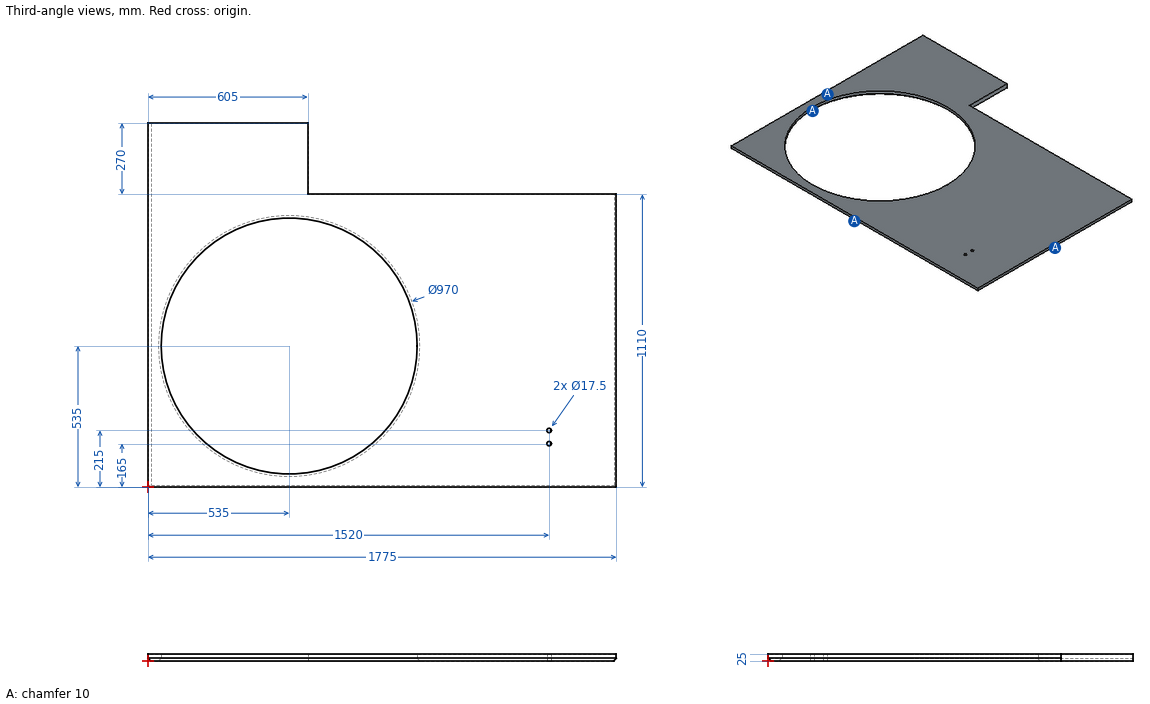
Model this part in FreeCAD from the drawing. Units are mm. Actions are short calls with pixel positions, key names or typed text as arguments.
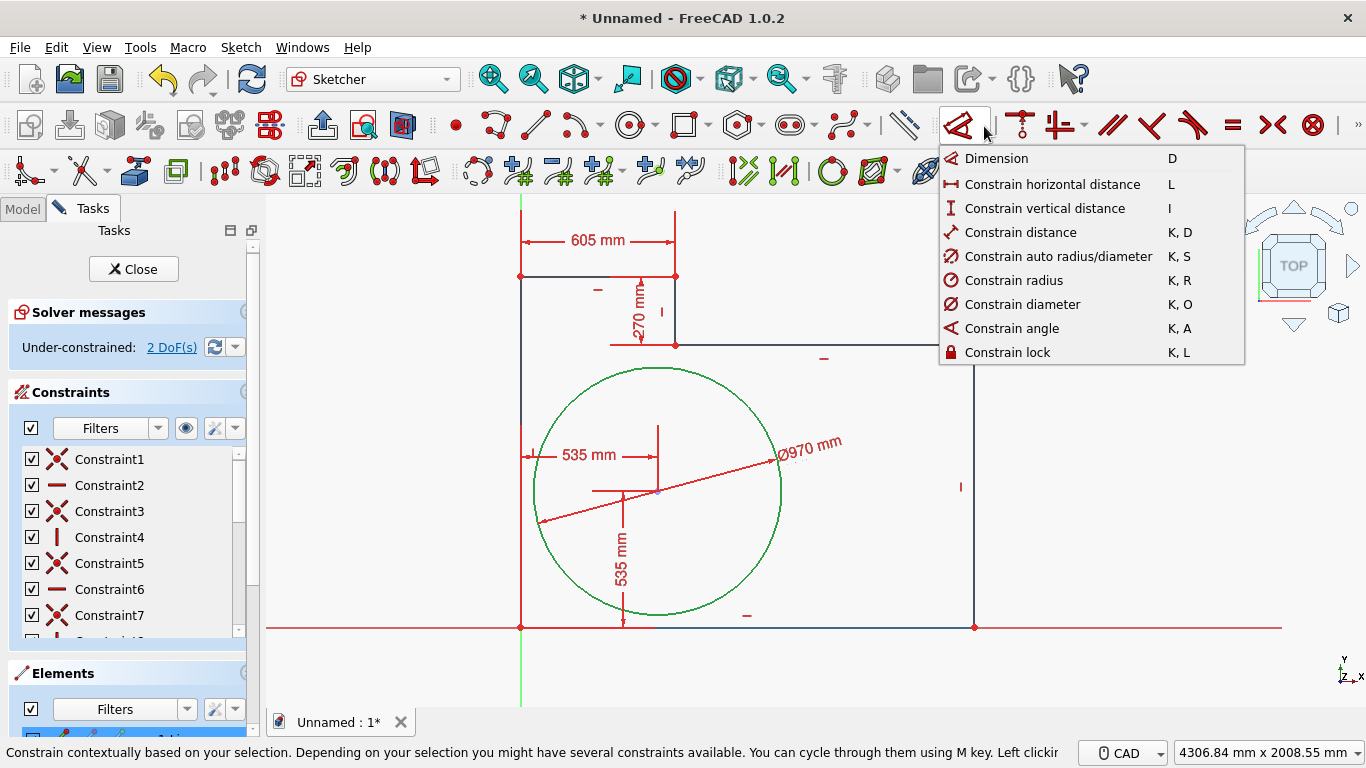
click(1092, 184)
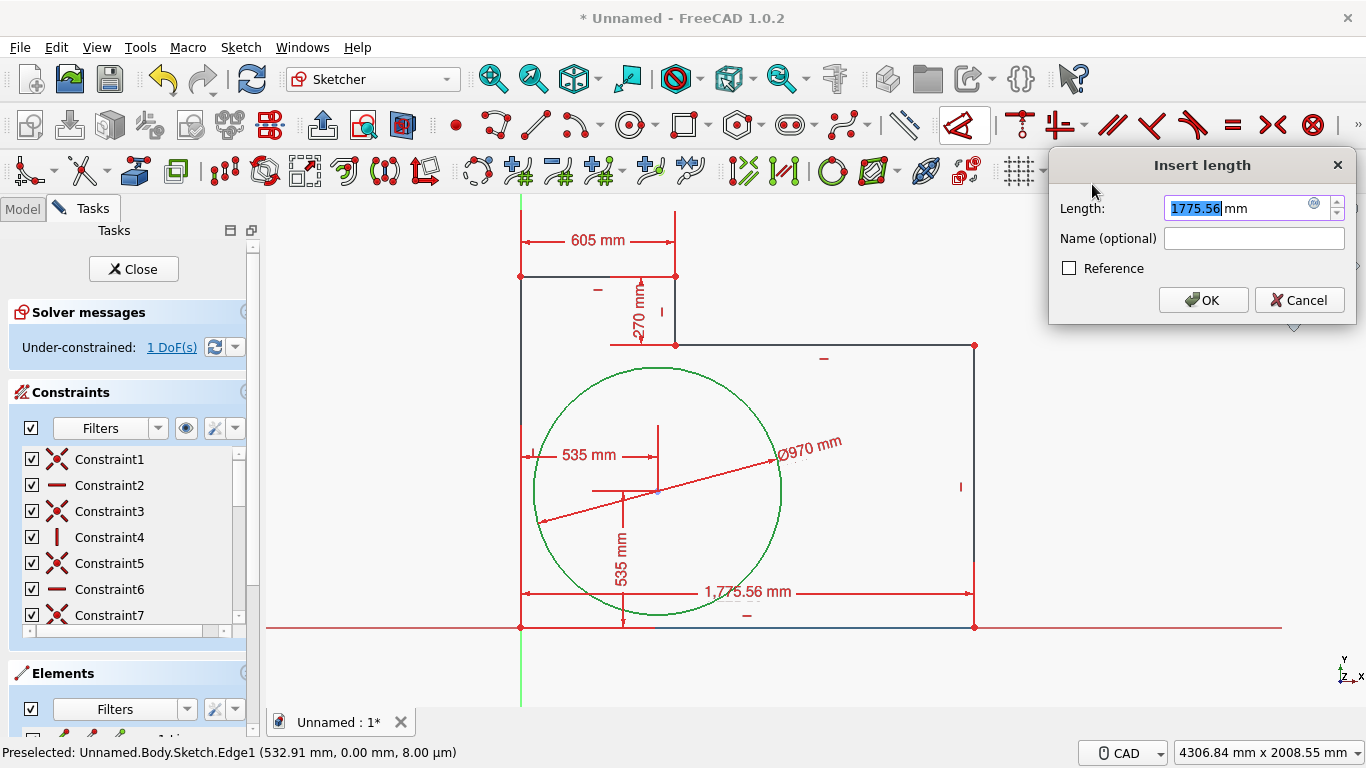
text(1775)
key(Return)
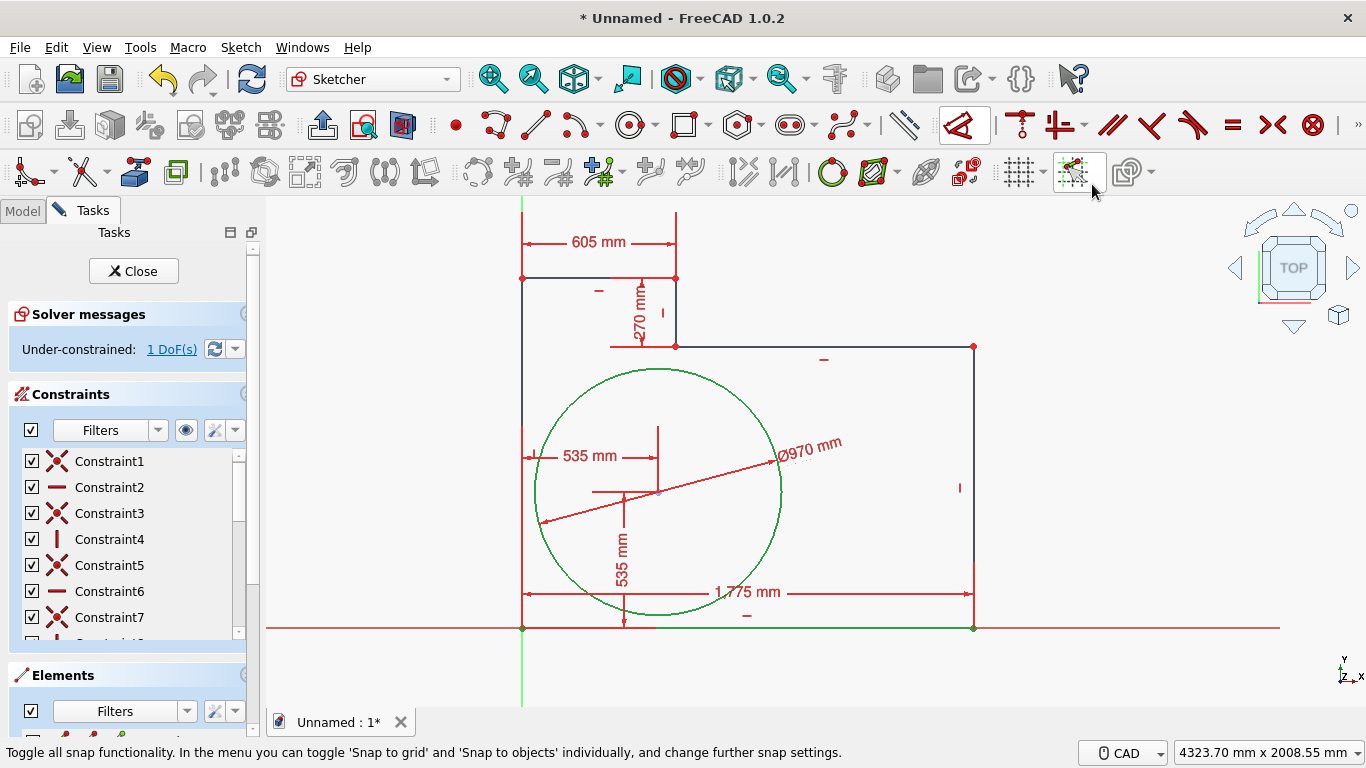
click(974, 544)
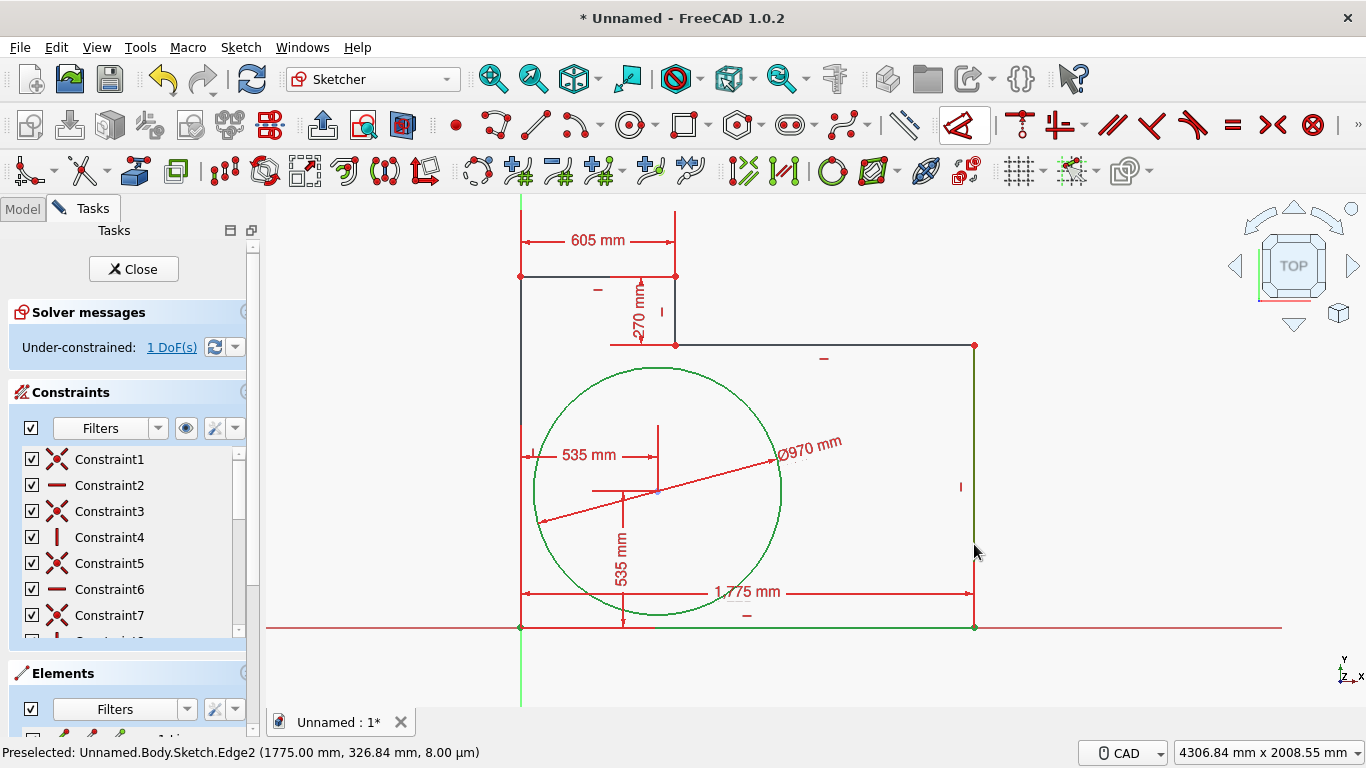
click(984, 126)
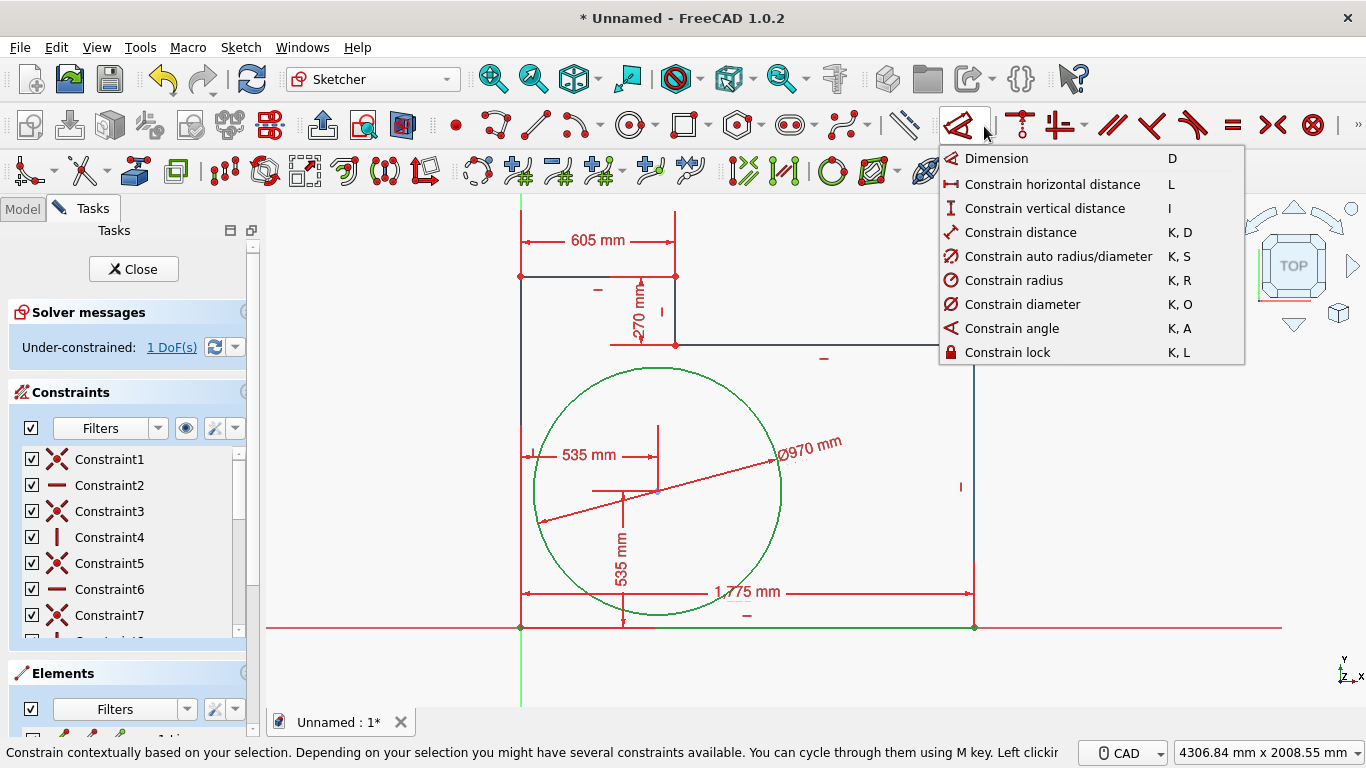
click(1092, 208)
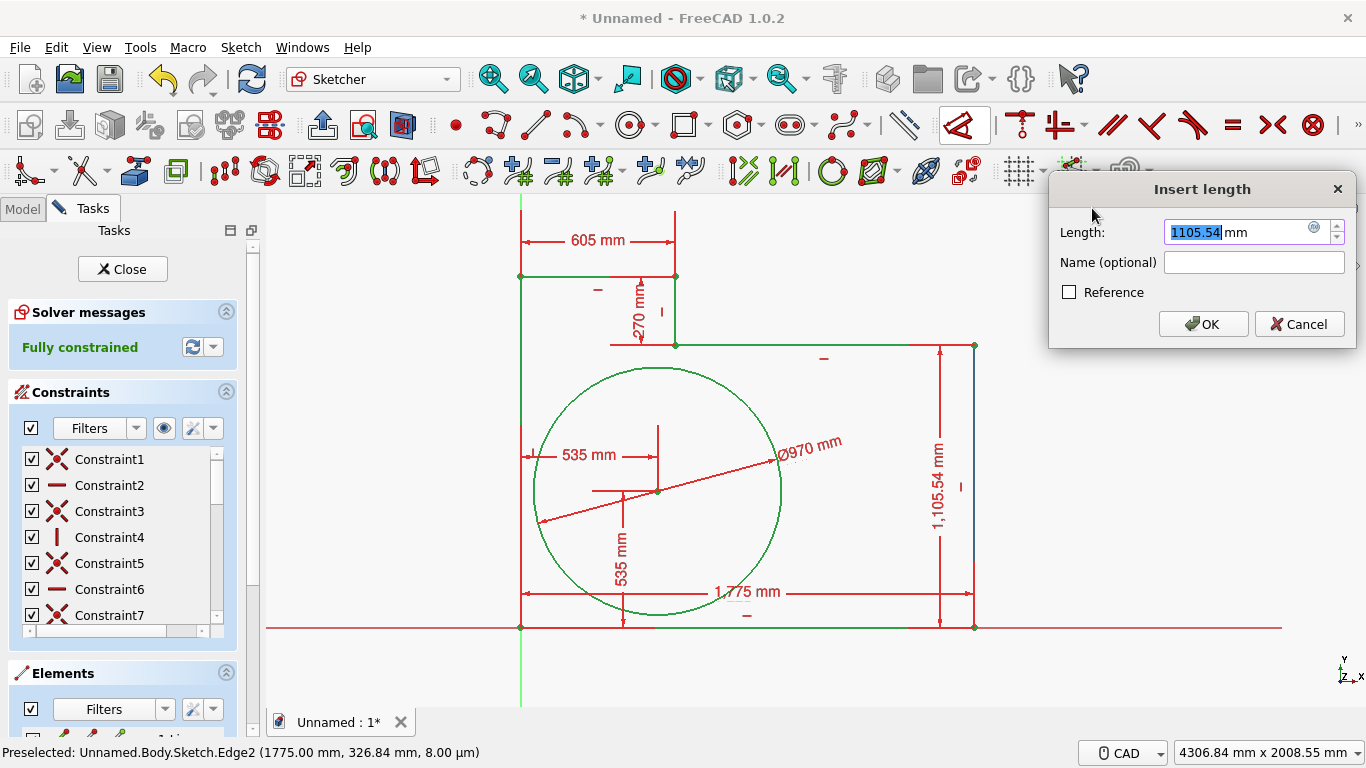
text(1110)
key(Return)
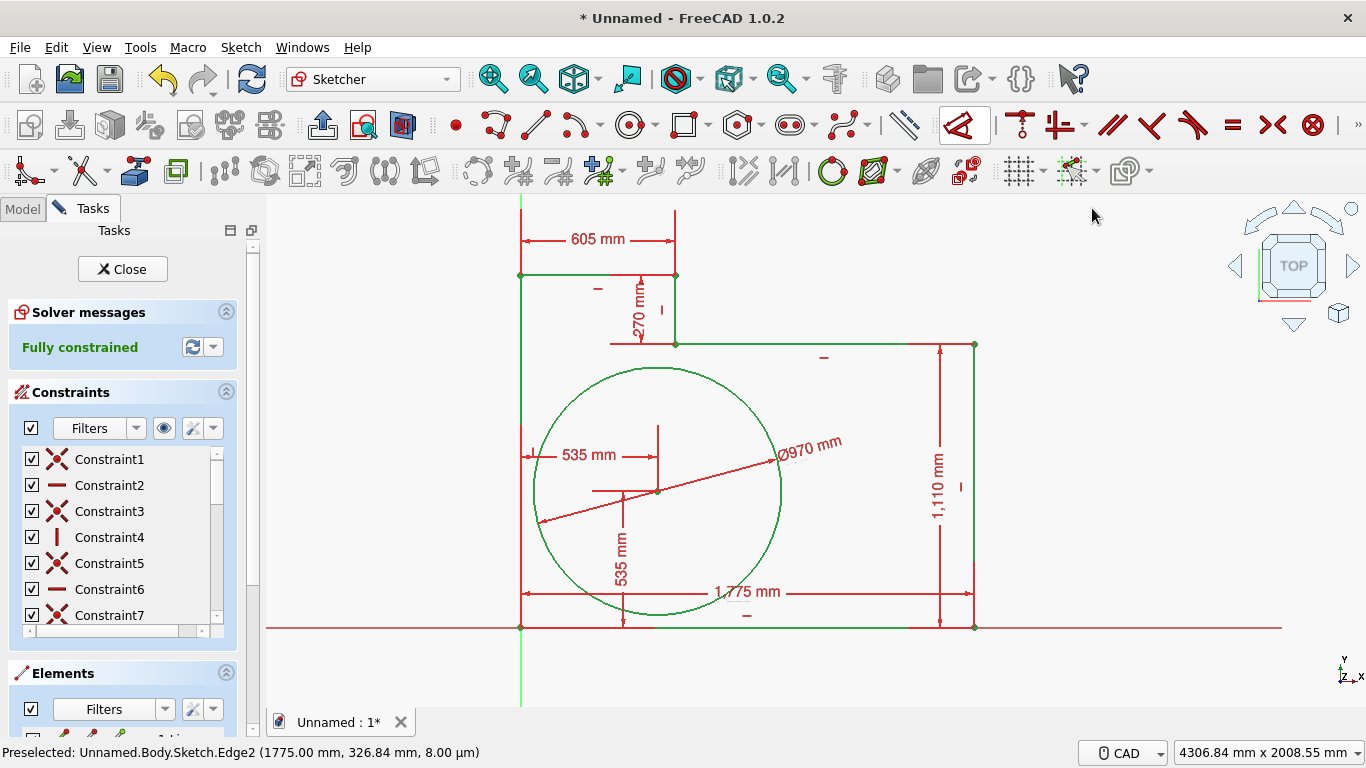
click(123, 269)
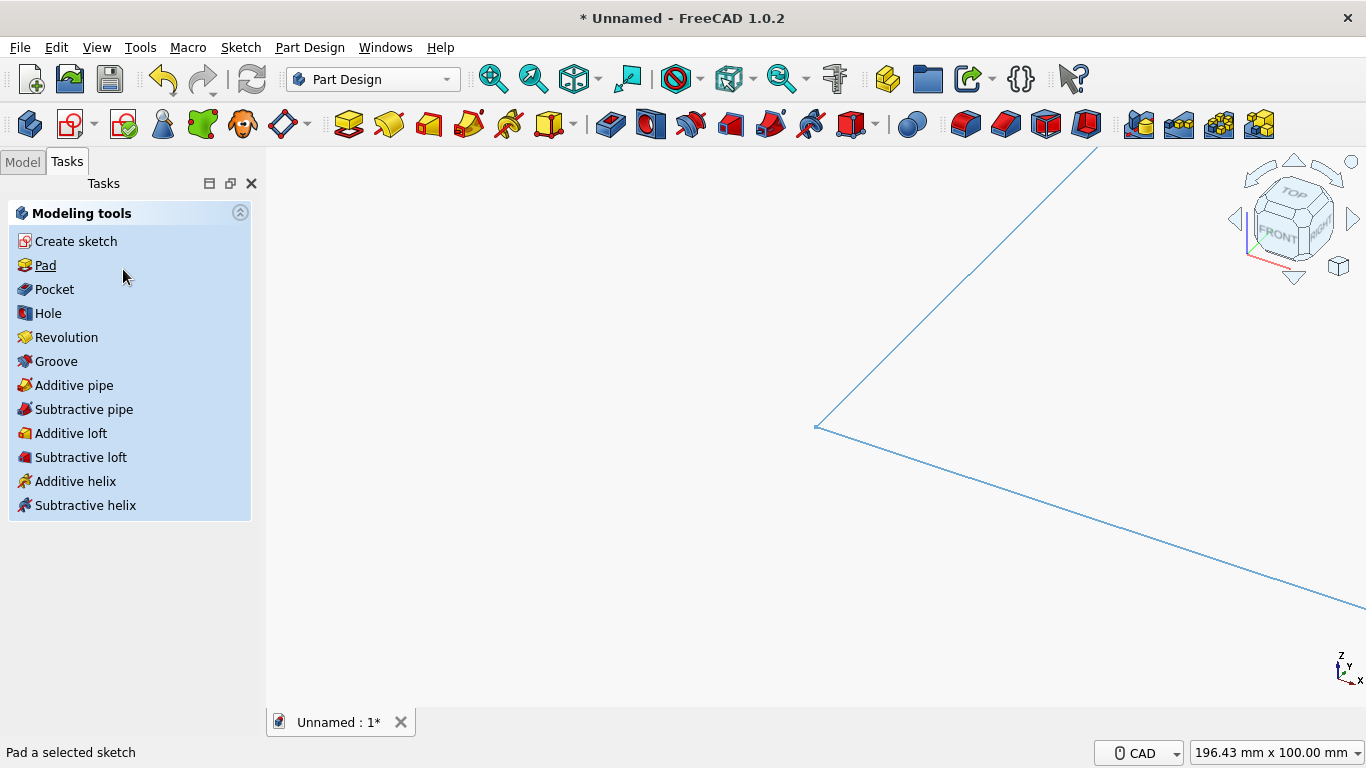
click(350, 124)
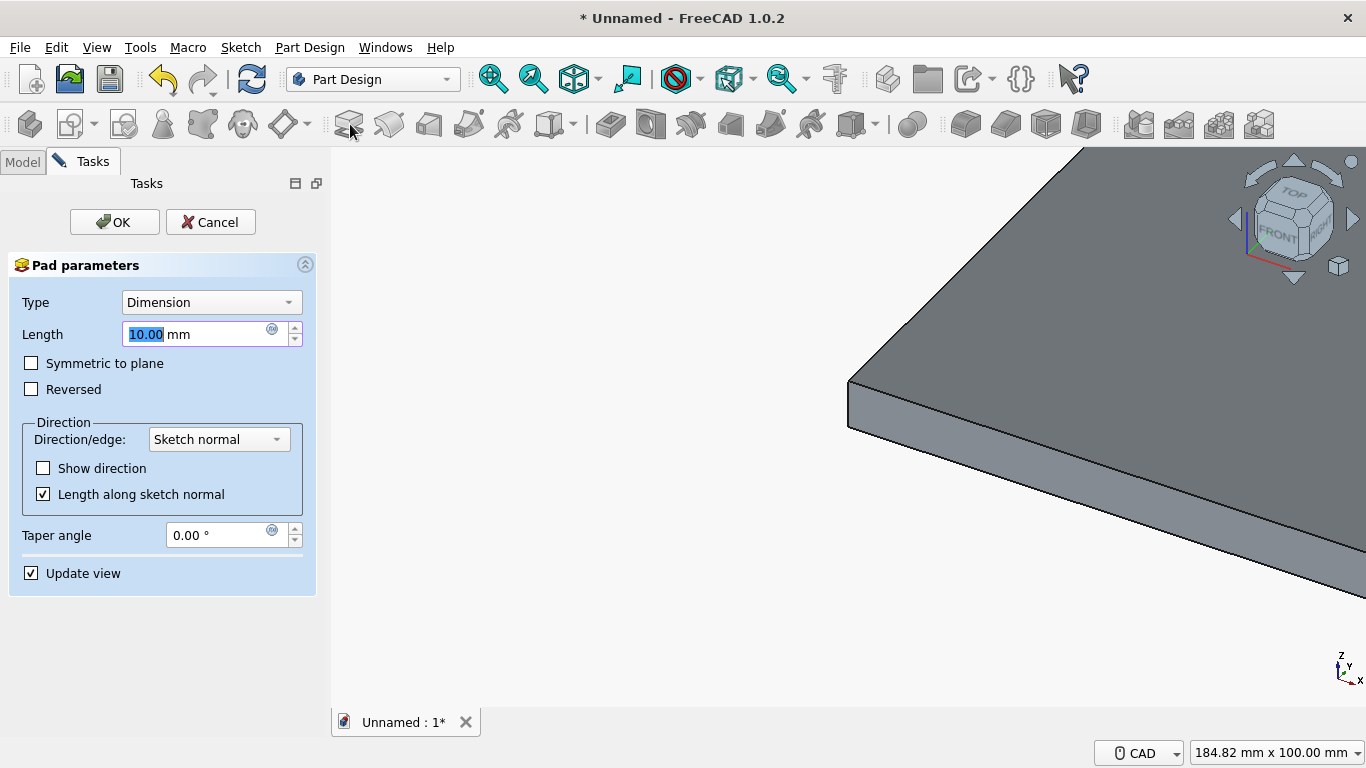
text(25)
key(Tab)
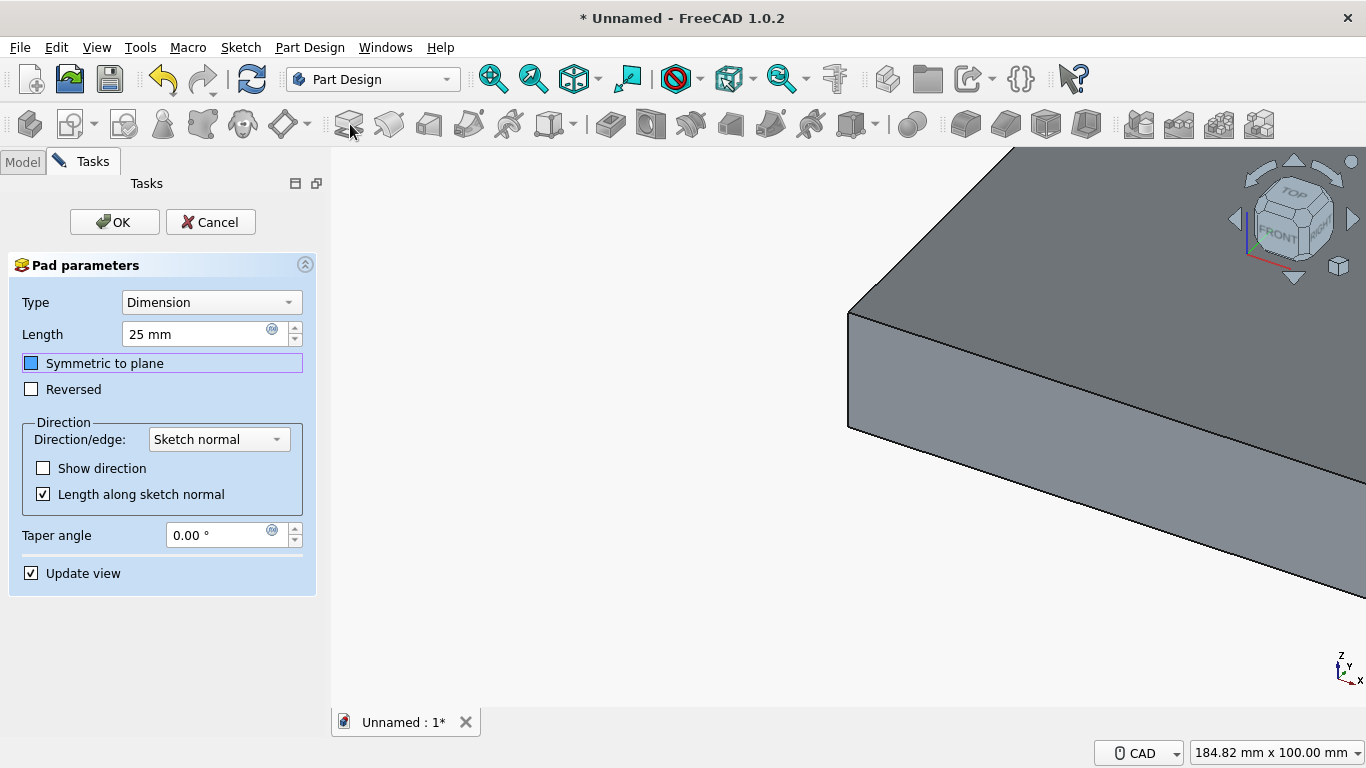
click(115, 222)